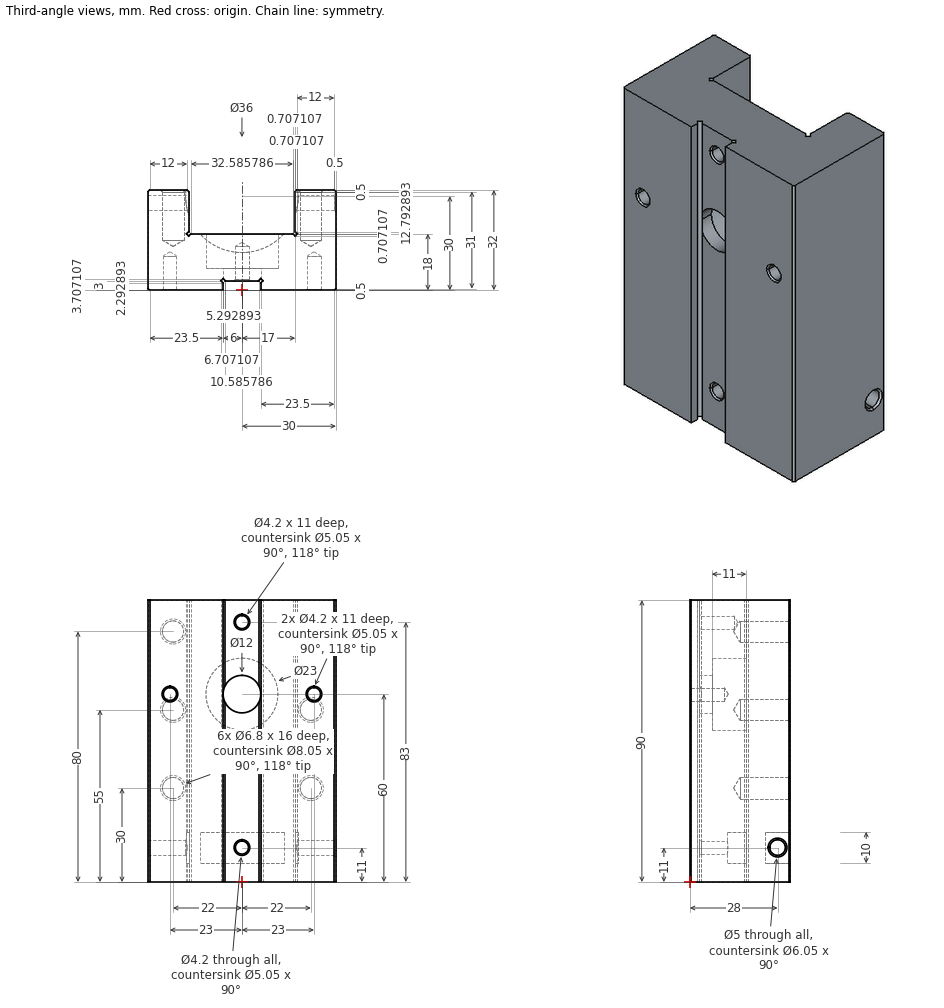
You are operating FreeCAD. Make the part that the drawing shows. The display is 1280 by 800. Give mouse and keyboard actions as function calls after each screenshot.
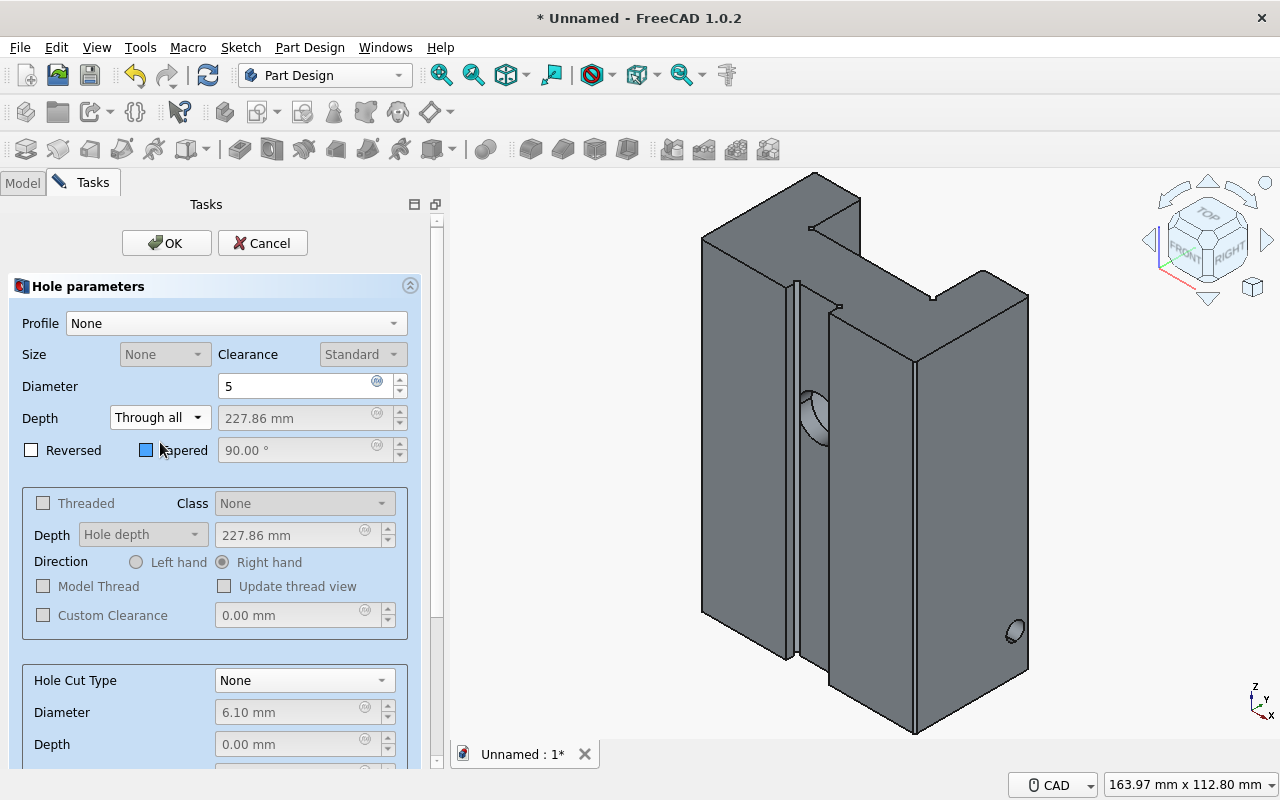
click(306, 680)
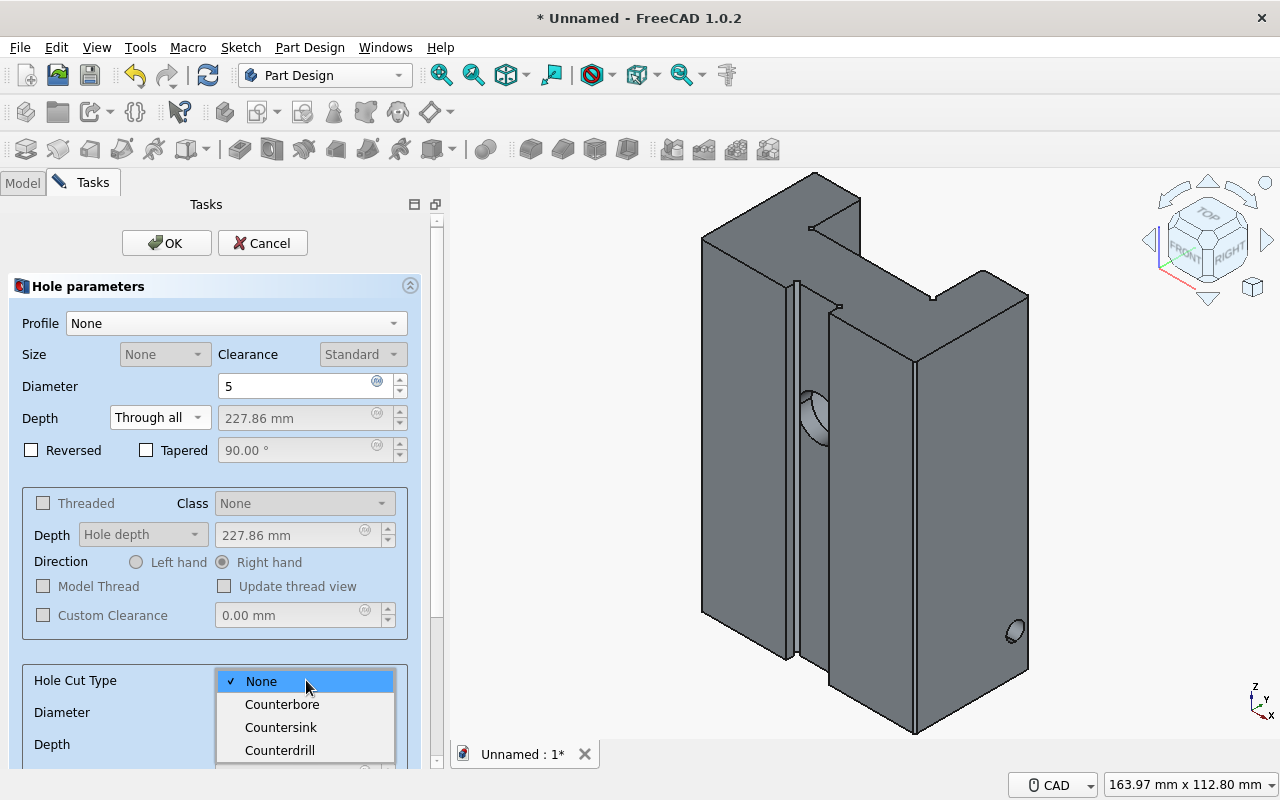
click(304, 728)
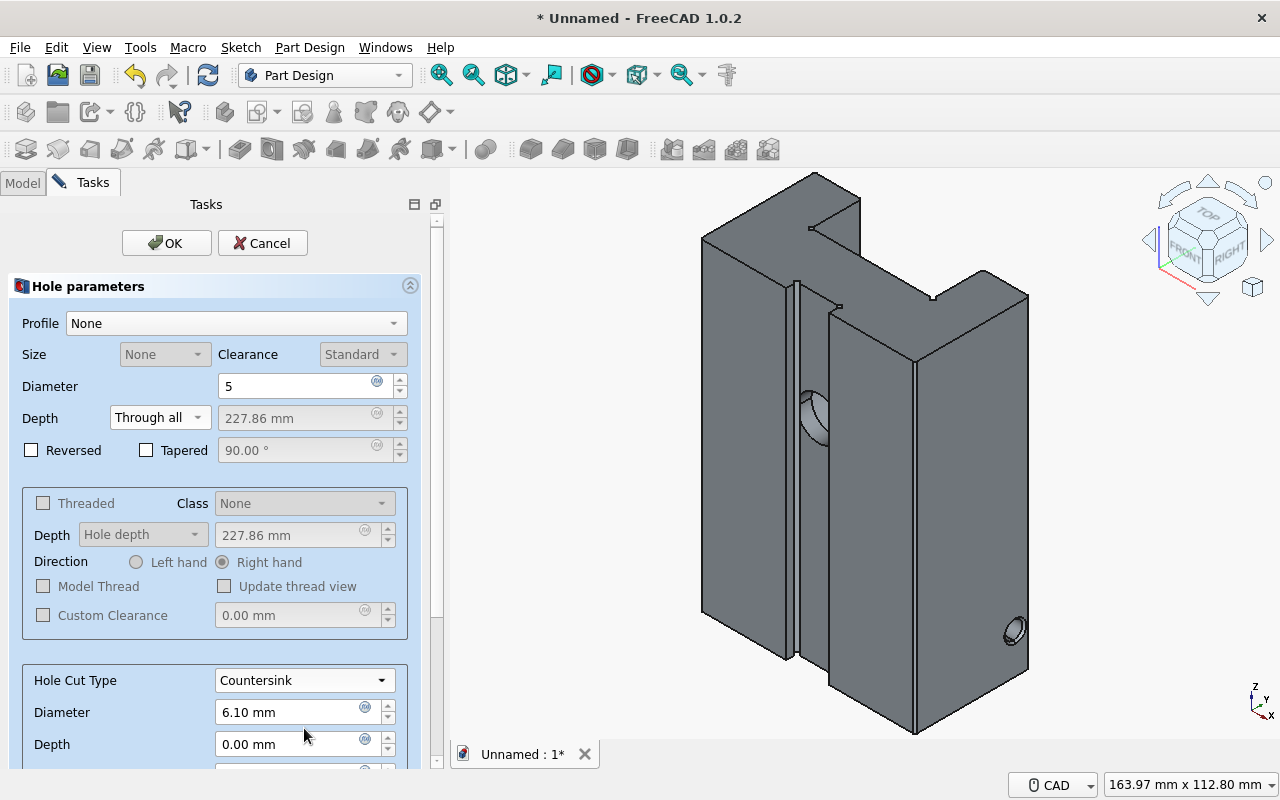
triple_click(298, 712)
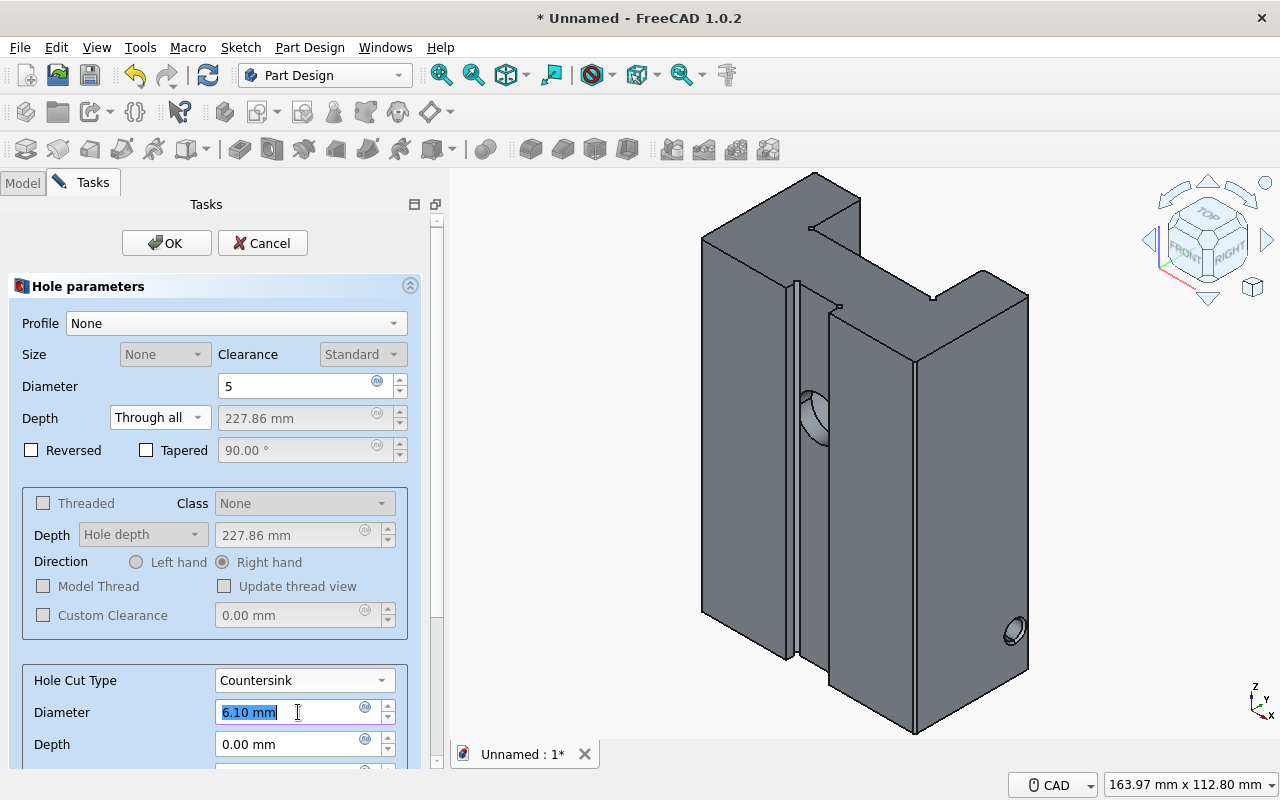
text(6.05)
key(Tab)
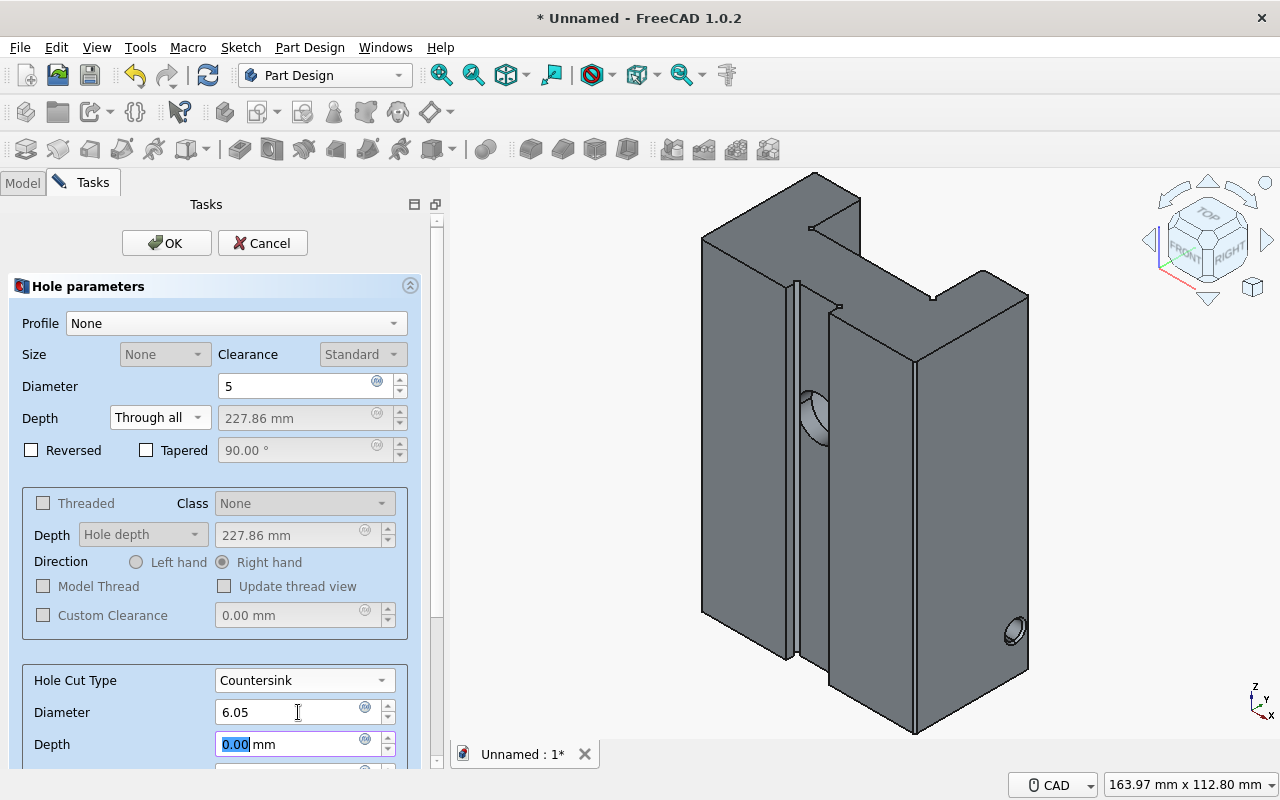
click(167, 243)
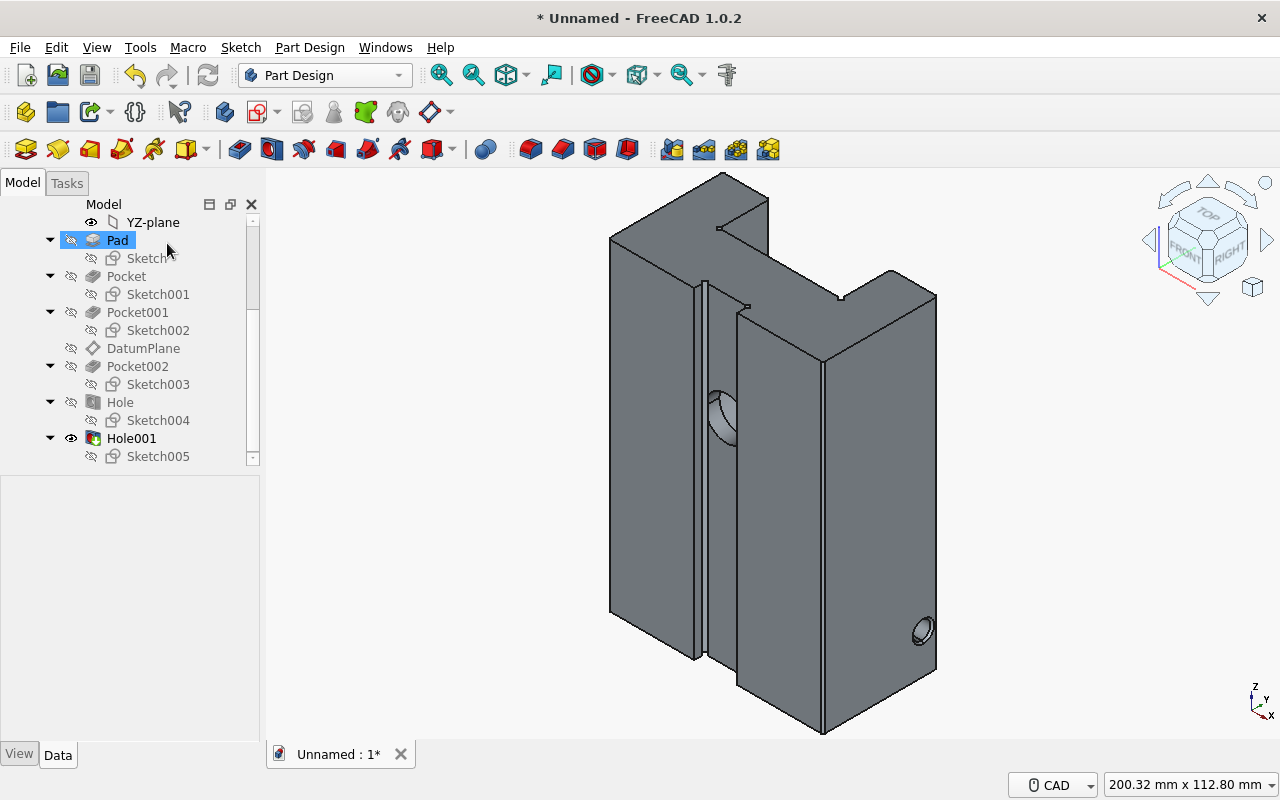
click(726, 480)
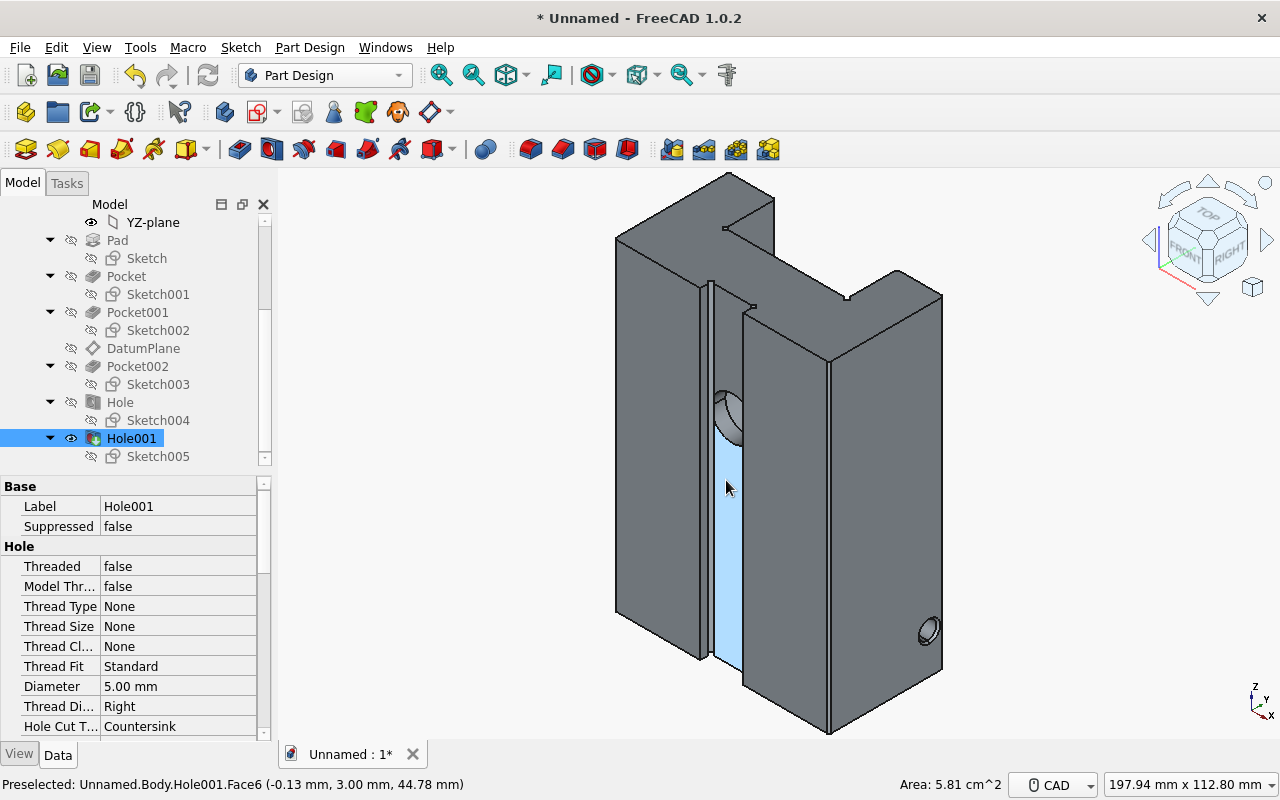
click(258, 112)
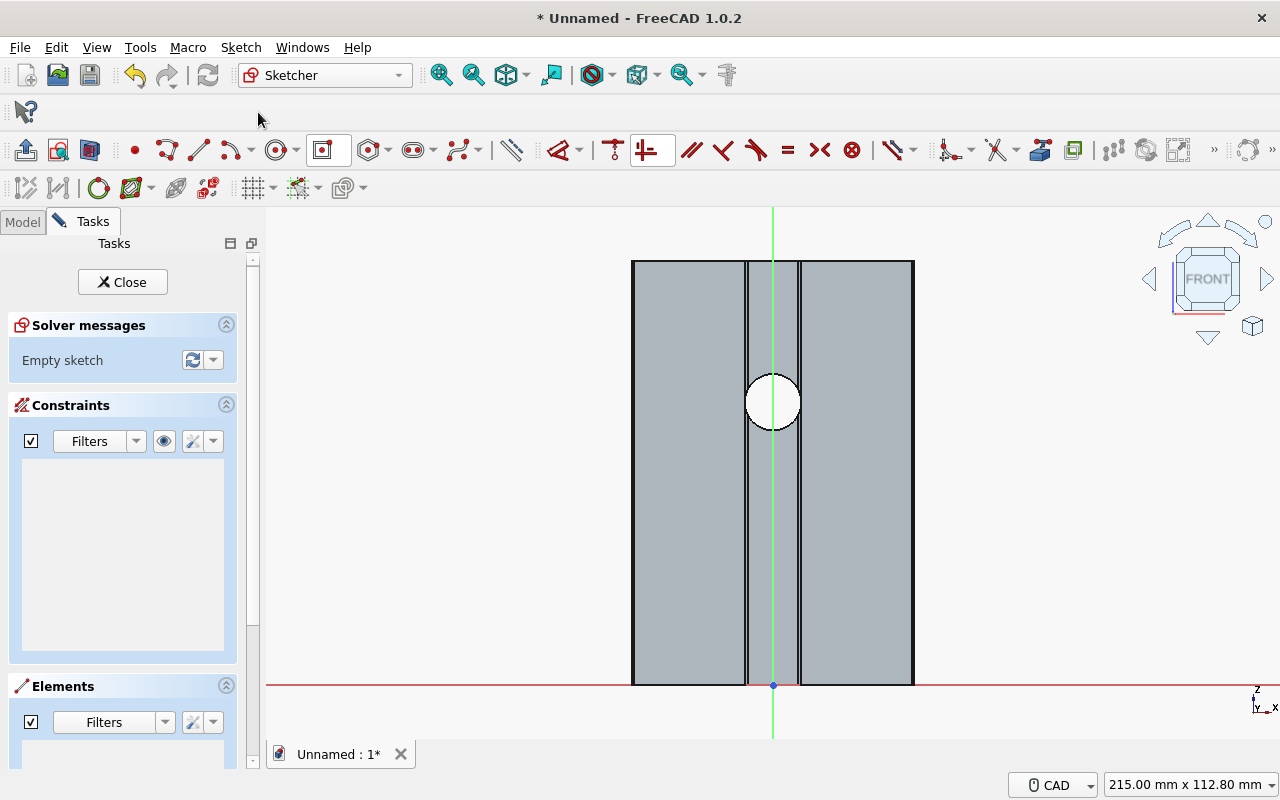
scroll(777, 644, up, 14)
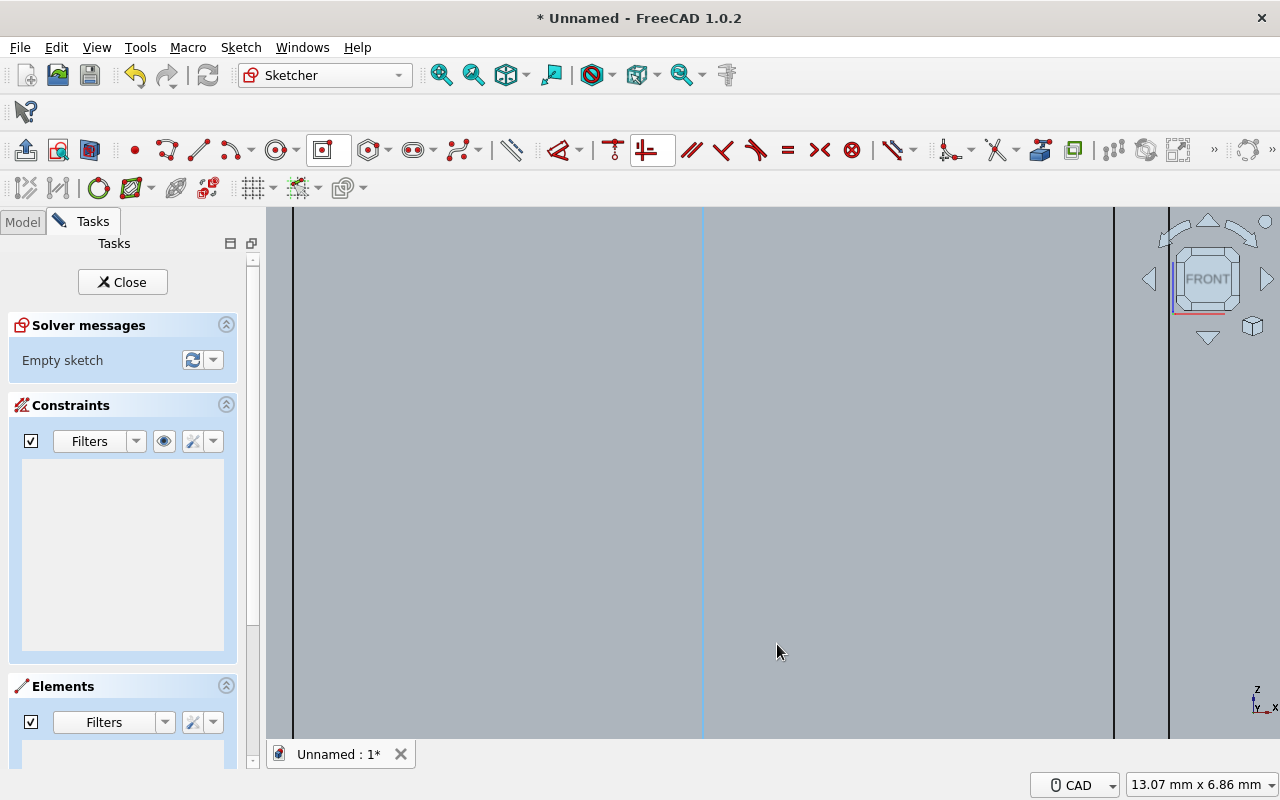
click(276, 150)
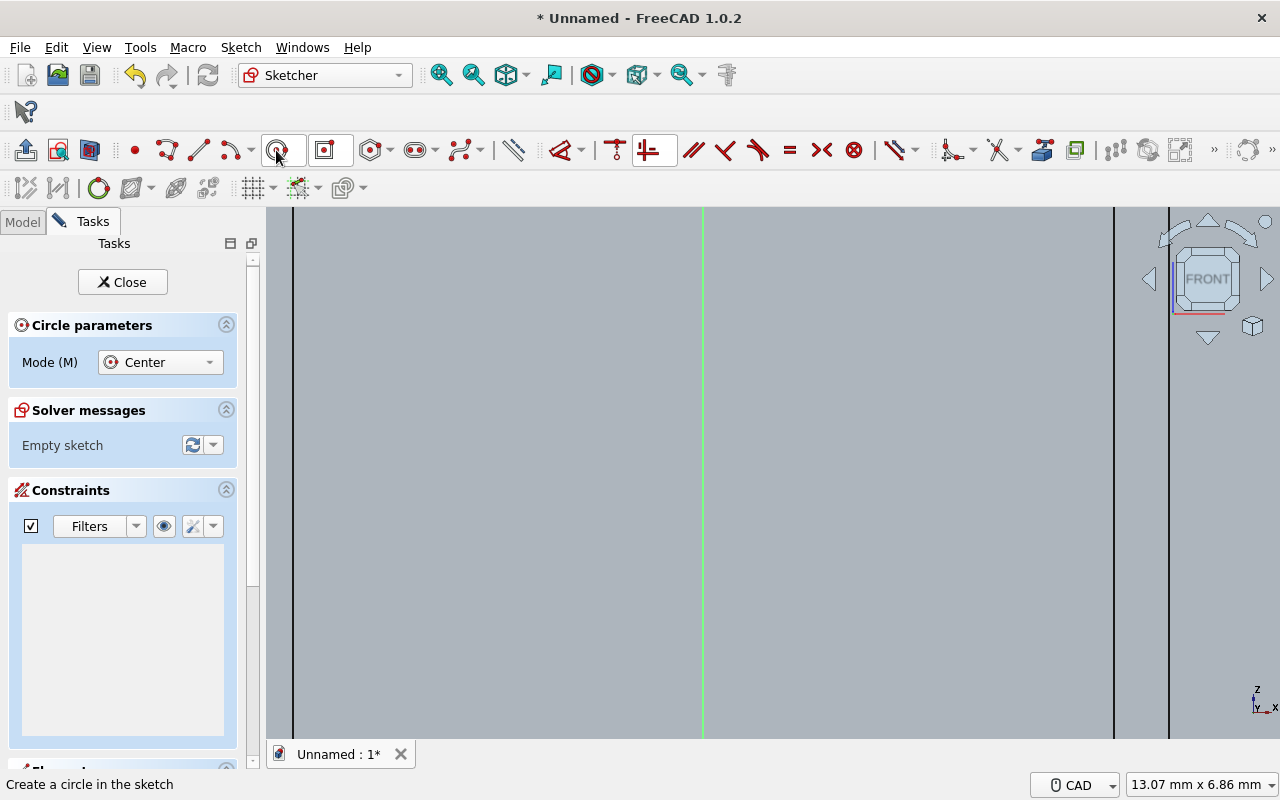
click(703, 456)
move(819, 341)